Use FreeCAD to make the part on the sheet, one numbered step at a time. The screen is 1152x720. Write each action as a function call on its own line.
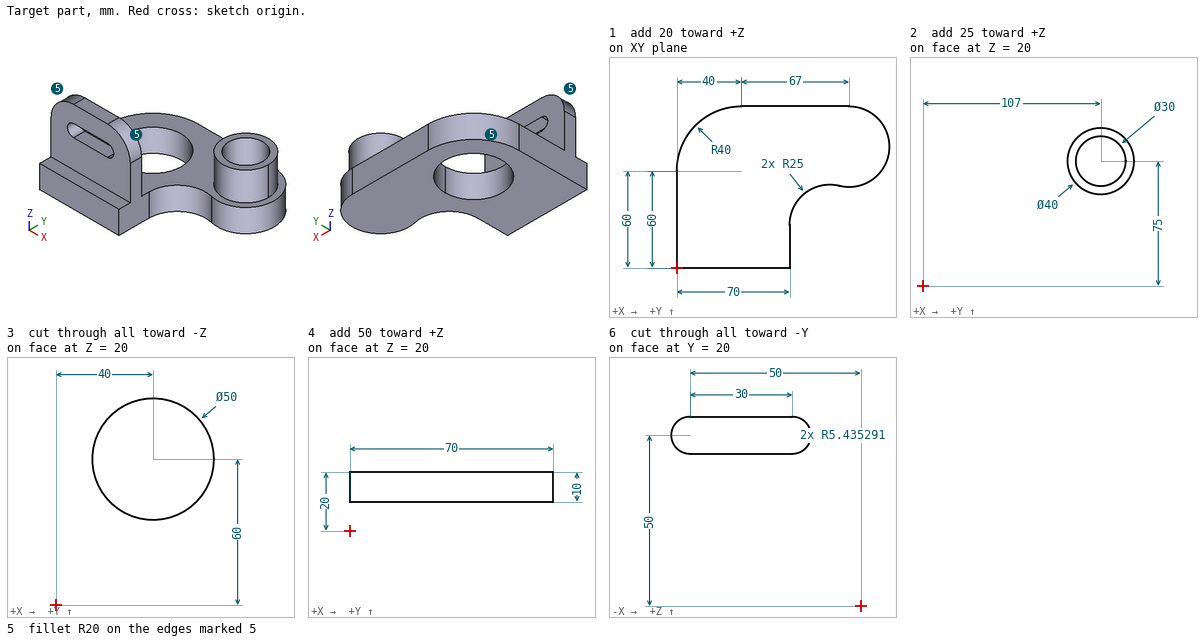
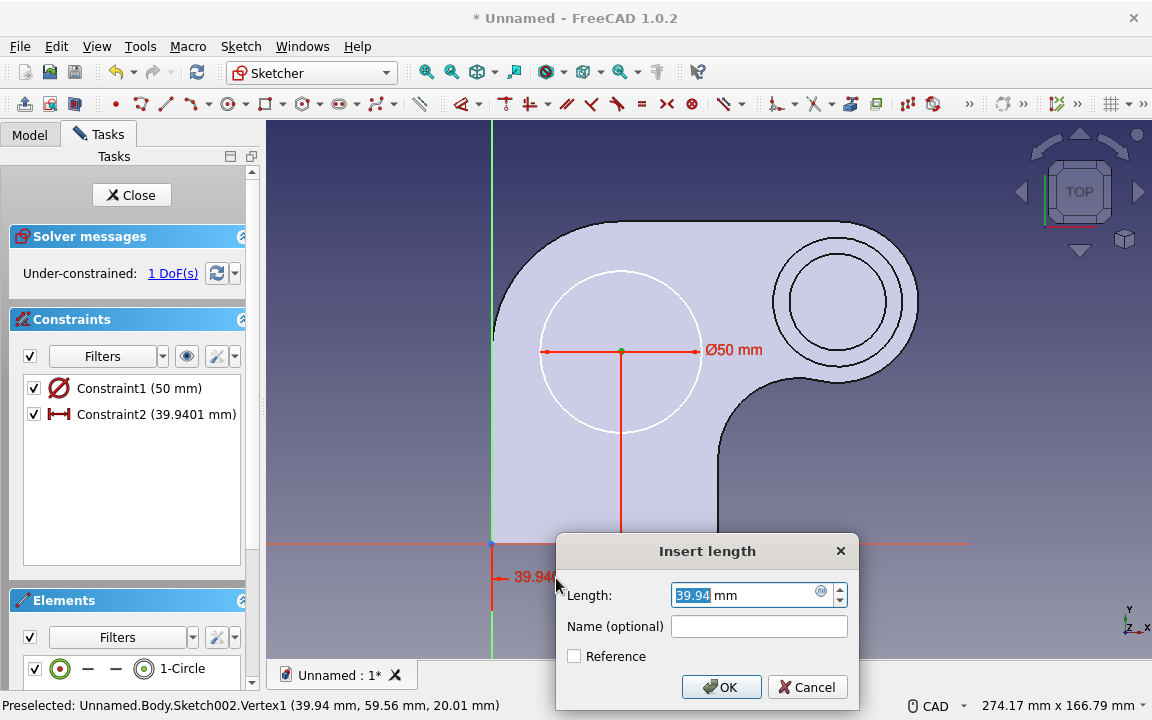
text(40)
key(Return)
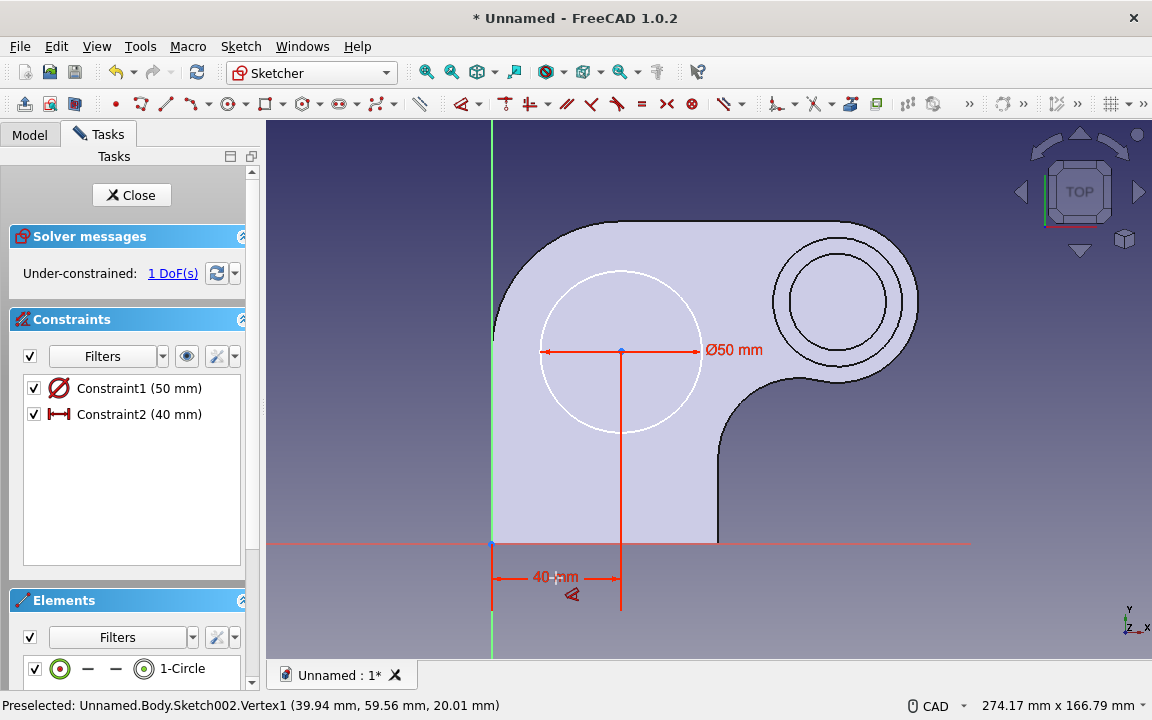
click(621, 352)
click(458, 448)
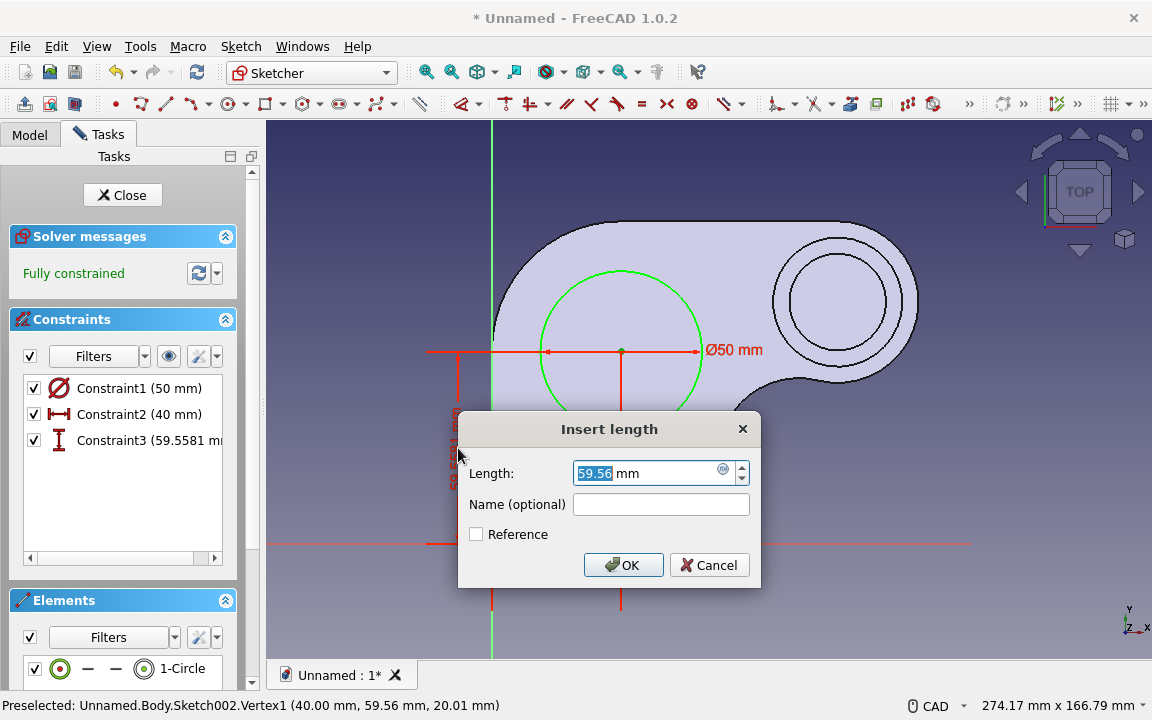
text(60)
key(Return)
key(Escape)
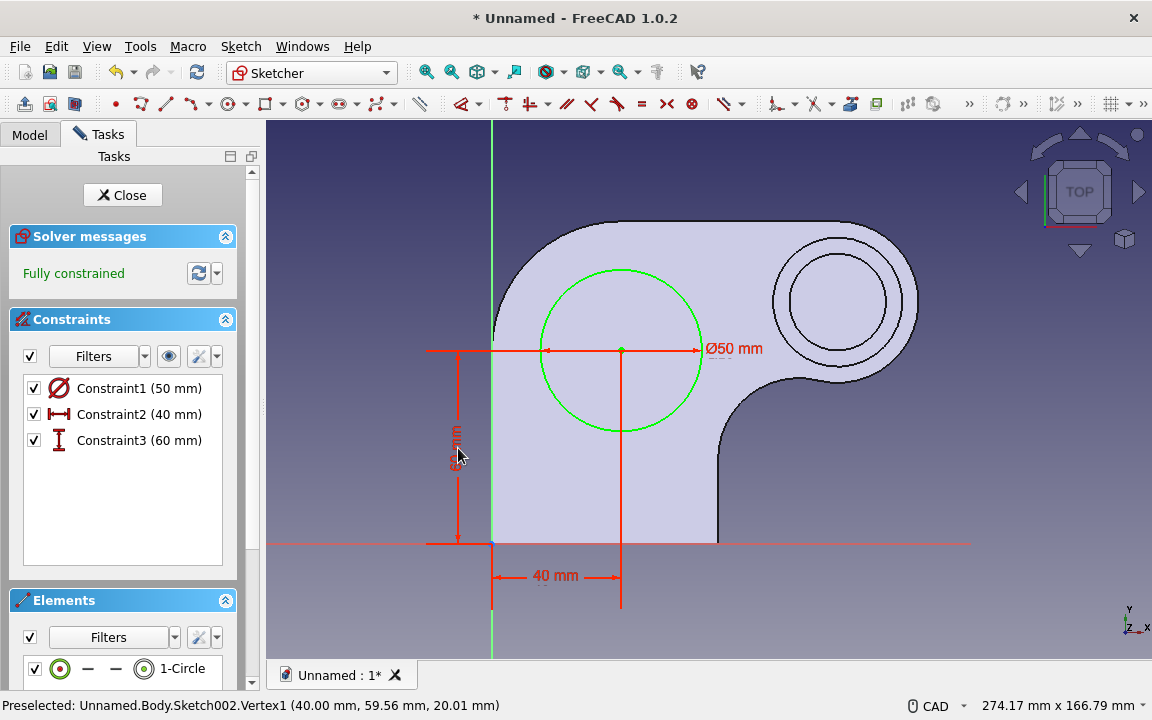
click(123, 195)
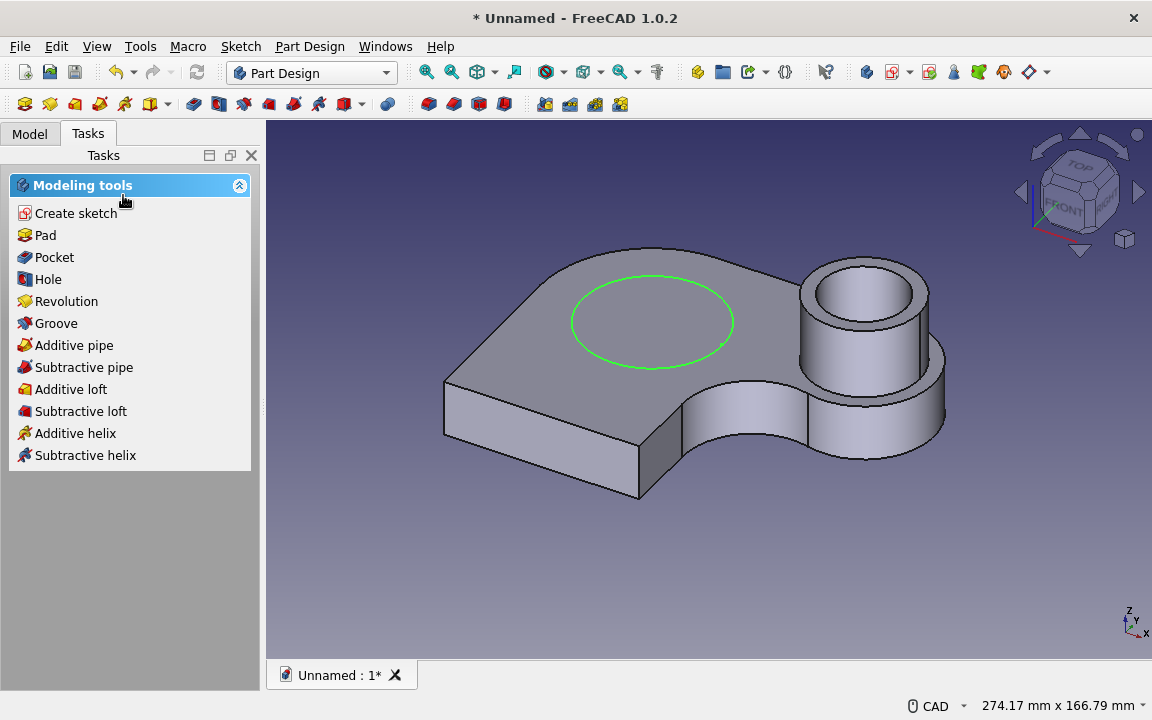
click(194, 104)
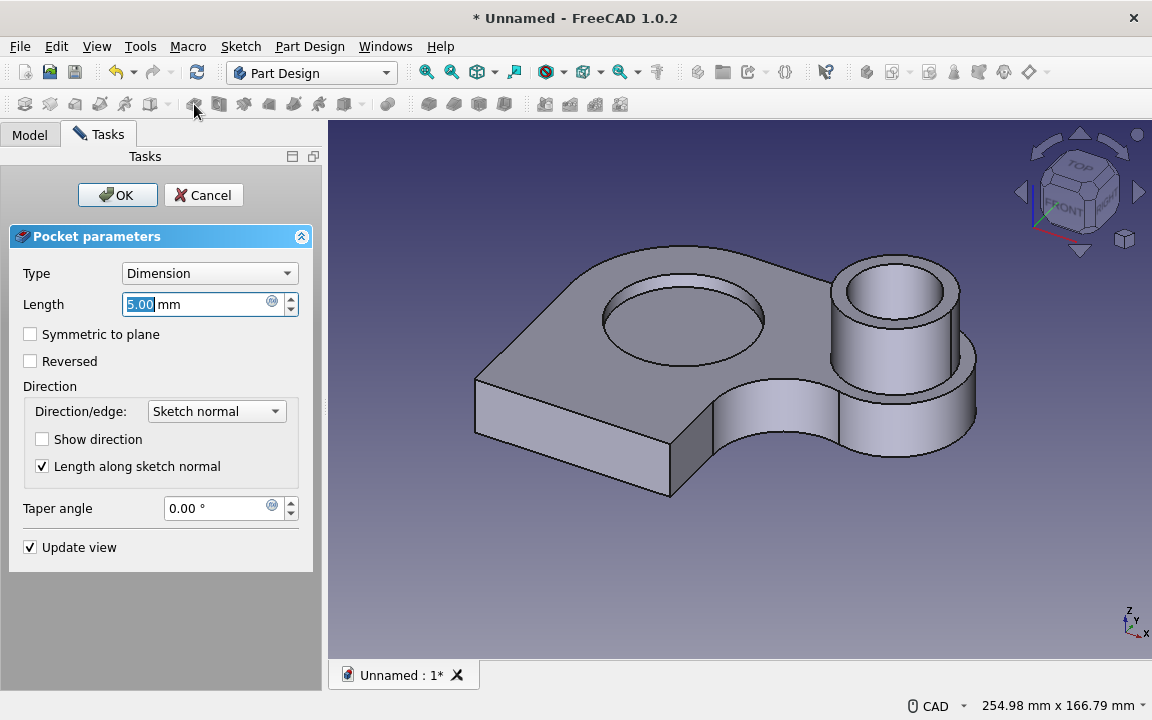
click(210, 274)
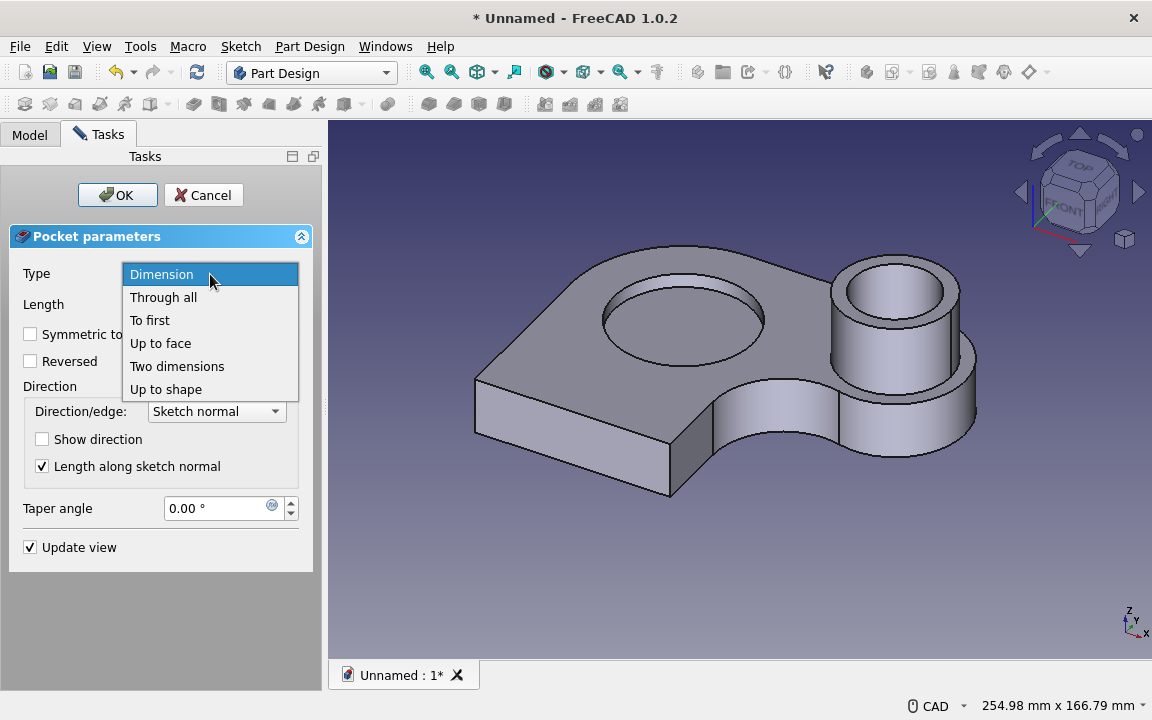
click(208, 298)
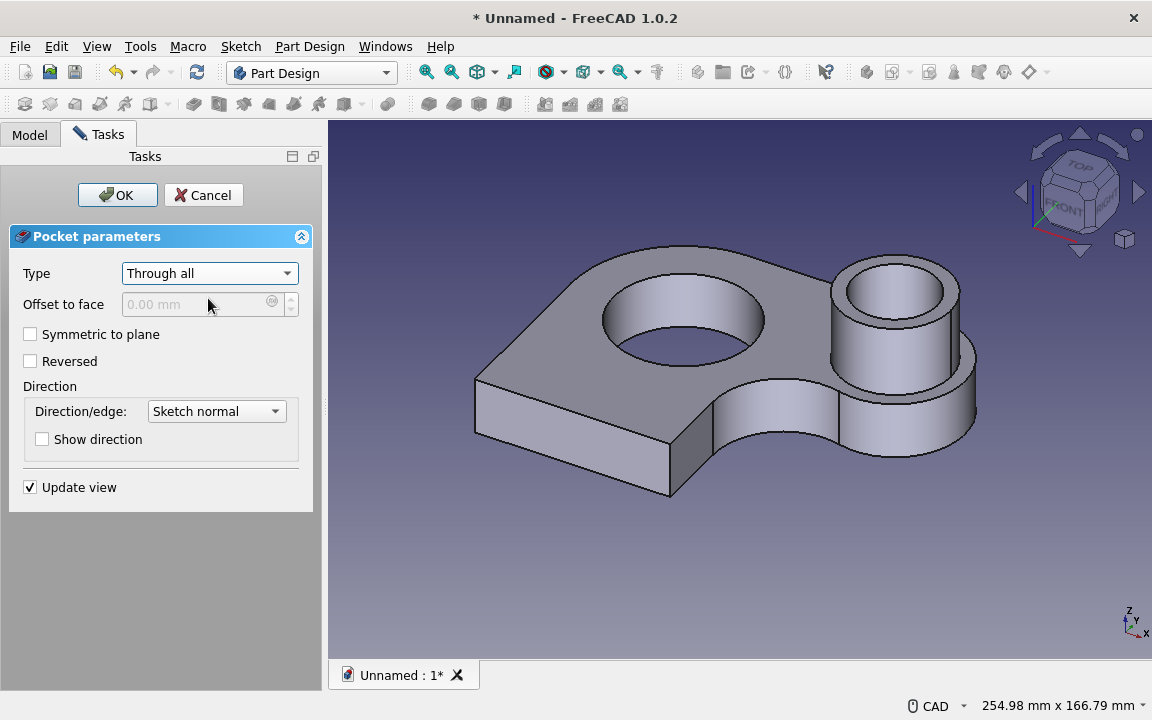
click(118, 195)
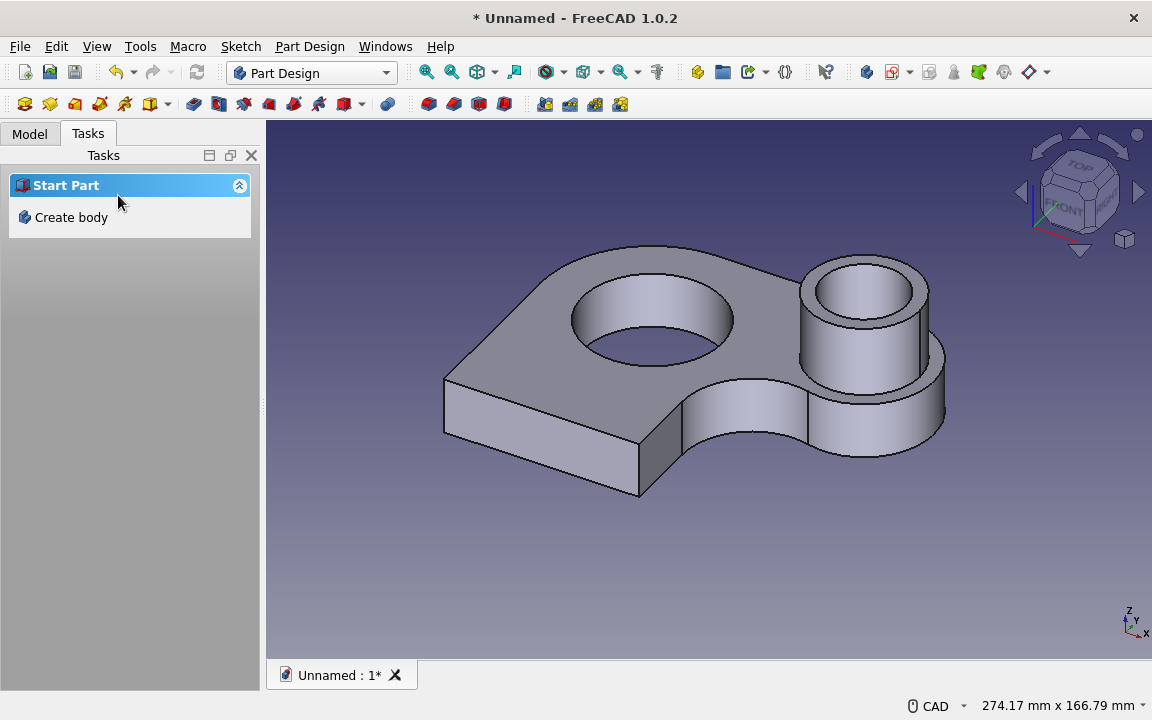
click(557, 370)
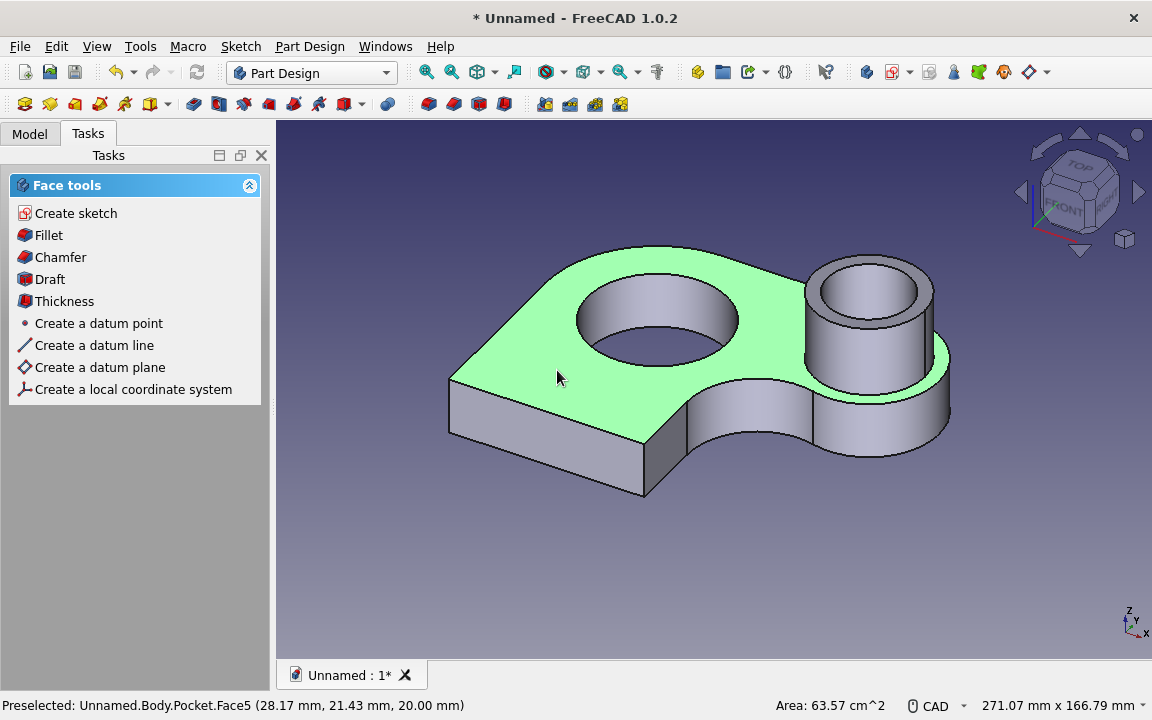
click(892, 72)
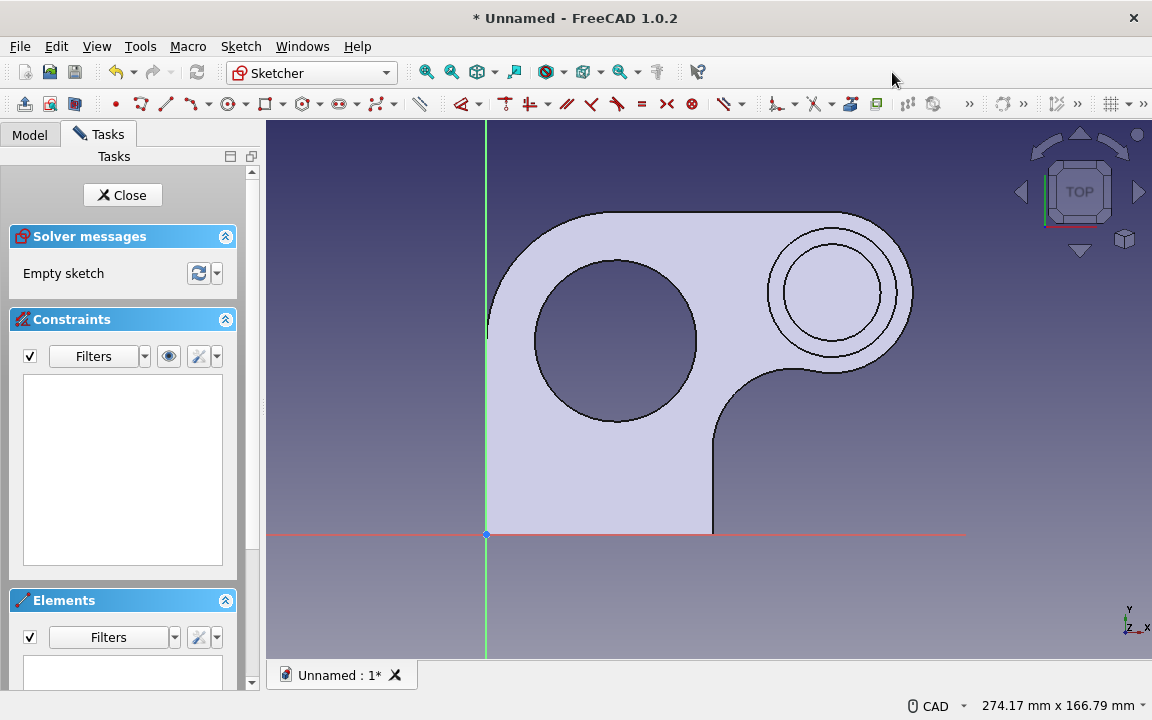
scroll(566, 595, up, 4)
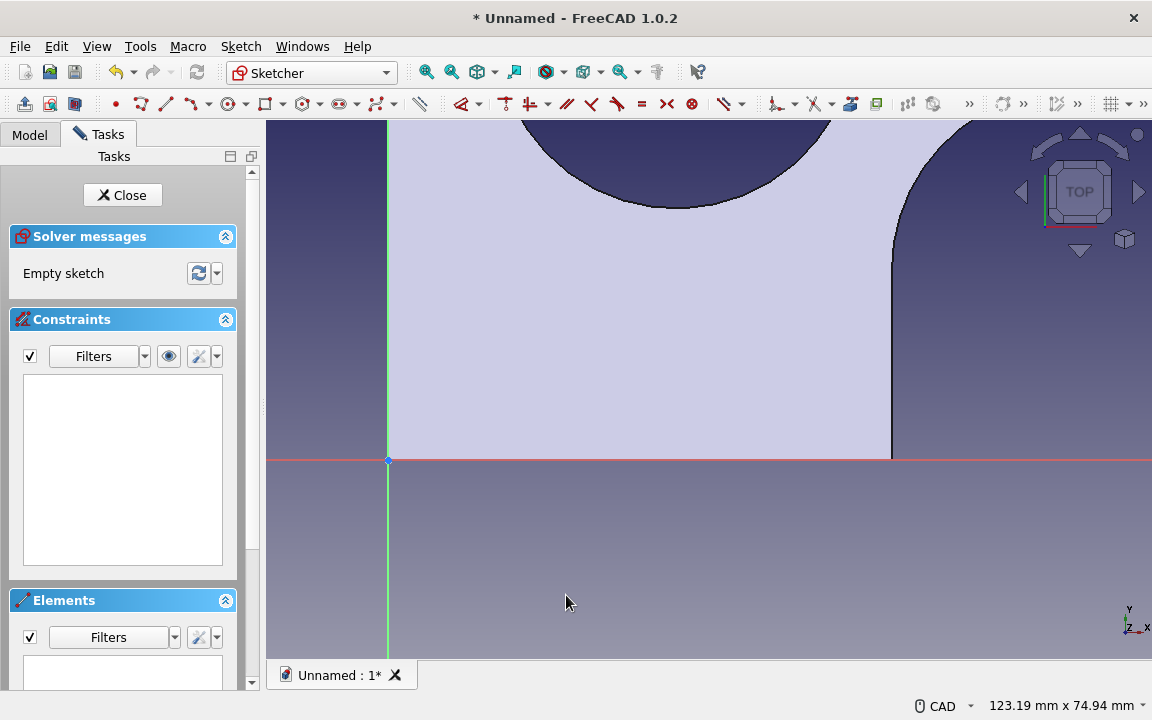
click(264, 104)